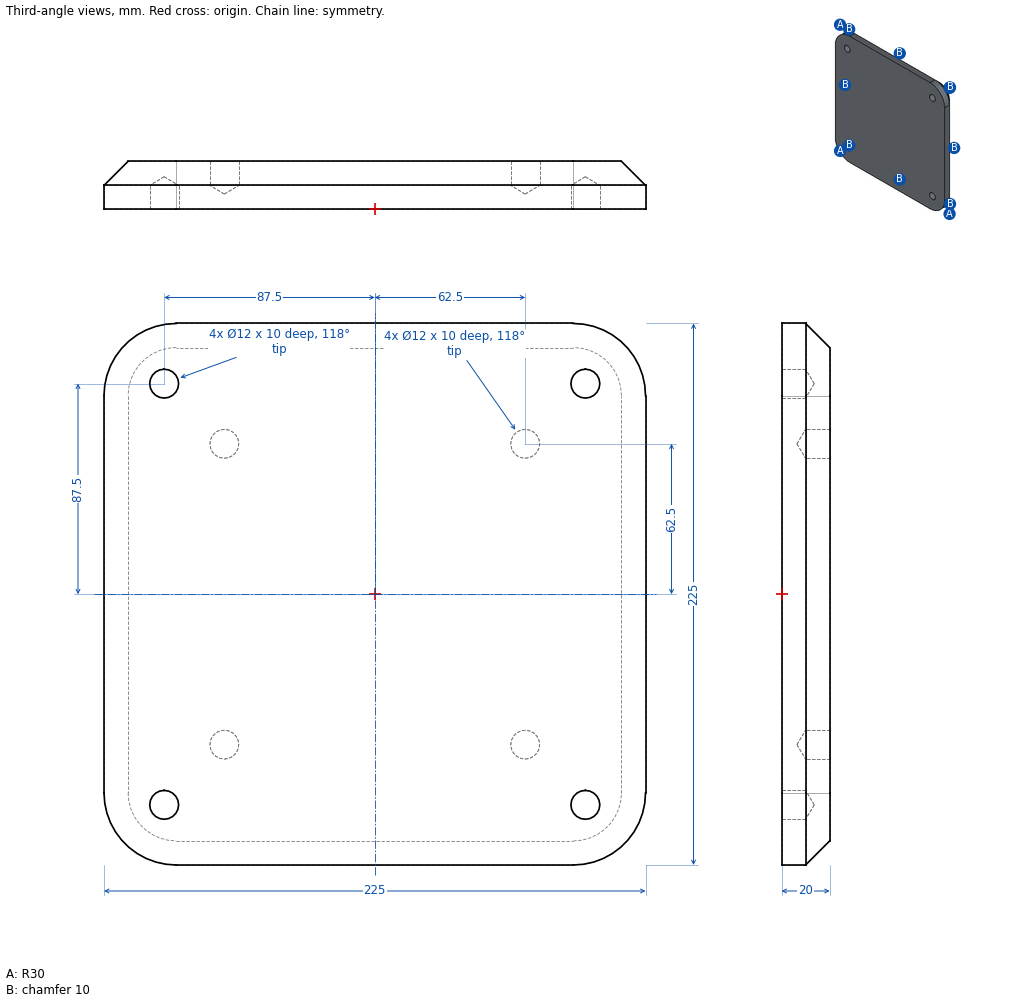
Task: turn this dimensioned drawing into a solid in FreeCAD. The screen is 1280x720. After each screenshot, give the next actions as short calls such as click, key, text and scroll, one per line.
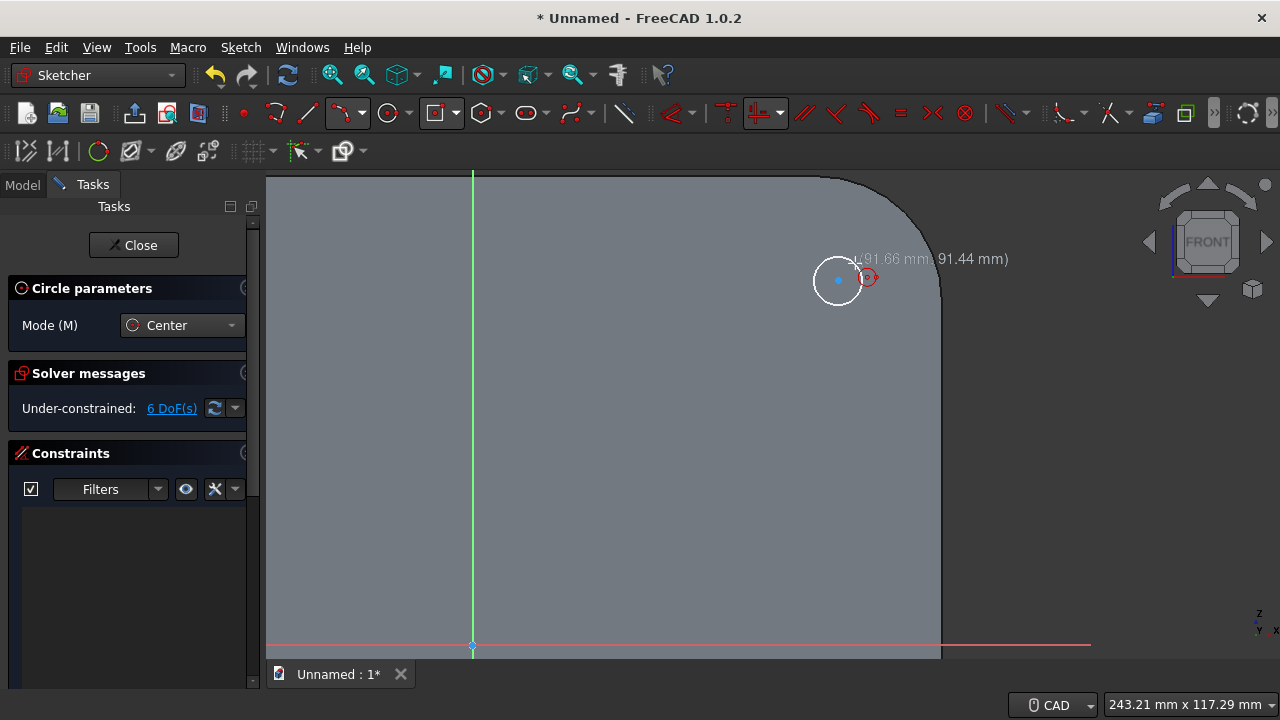
scroll(839, 280, down, 5)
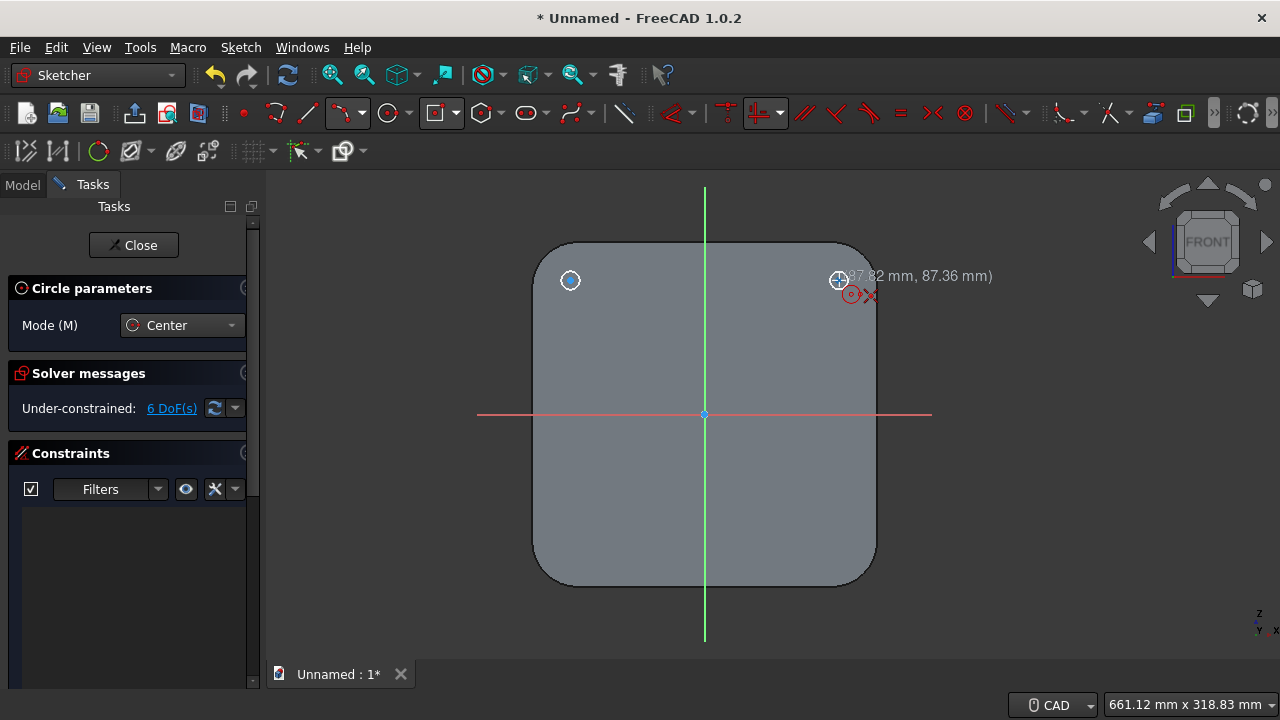
scroll(839, 549, up, 5)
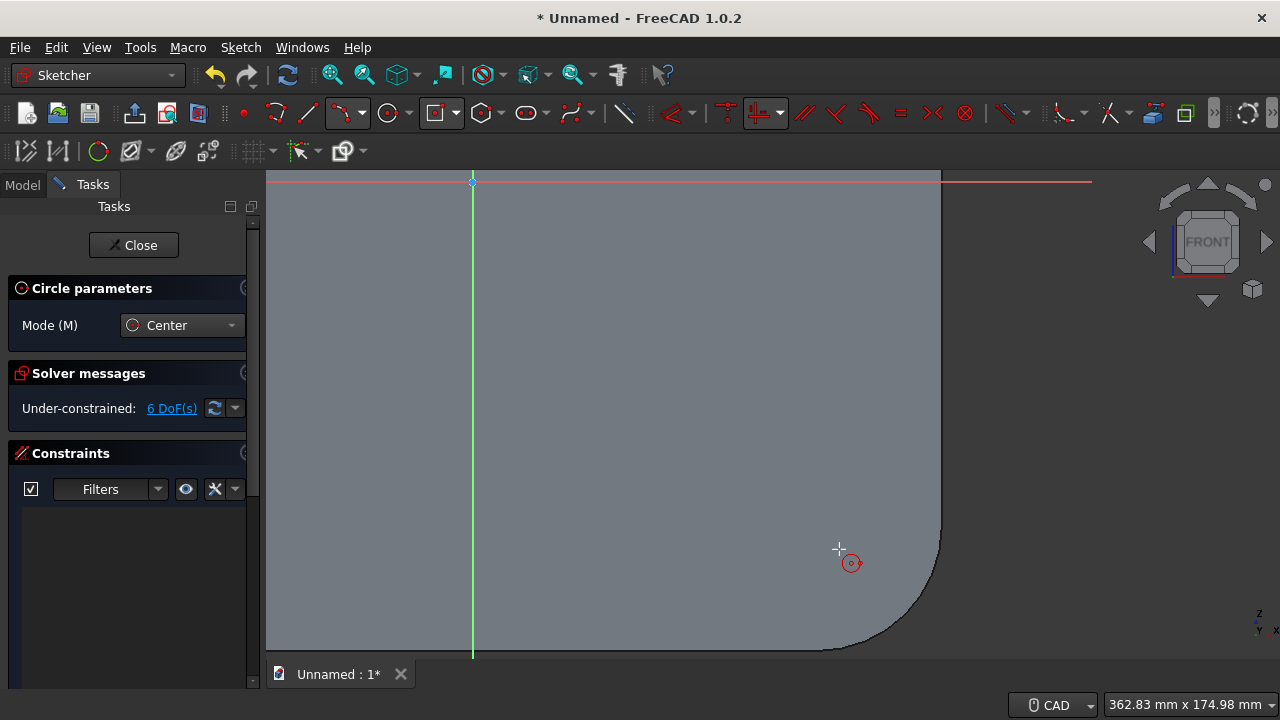
click(838, 547)
click(855, 529)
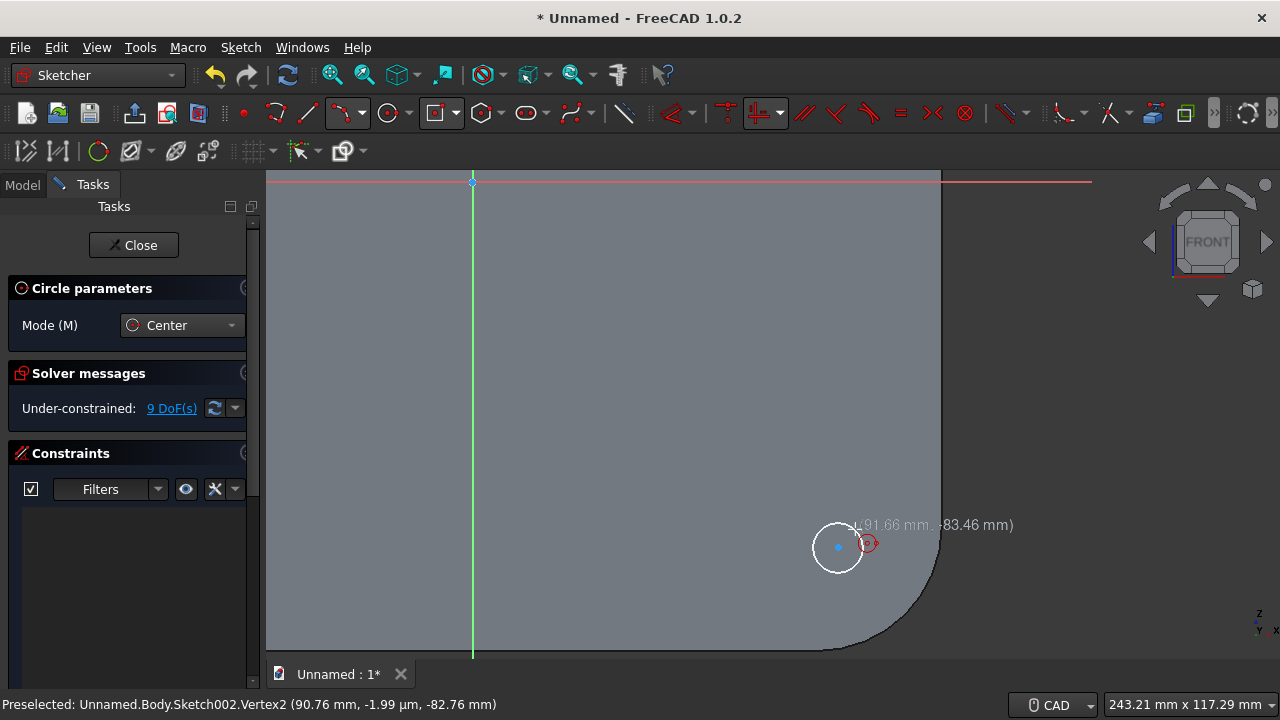
scroll(839, 550, down, 5)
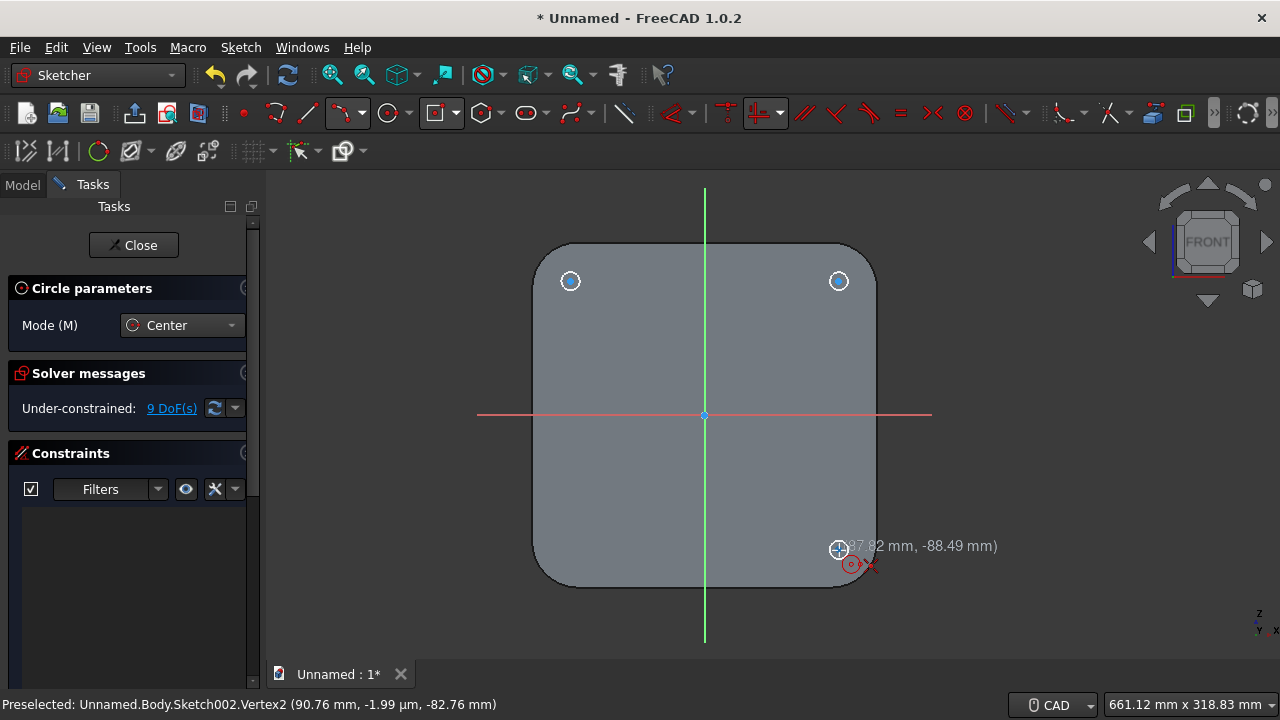
scroll(570, 549, up, 5)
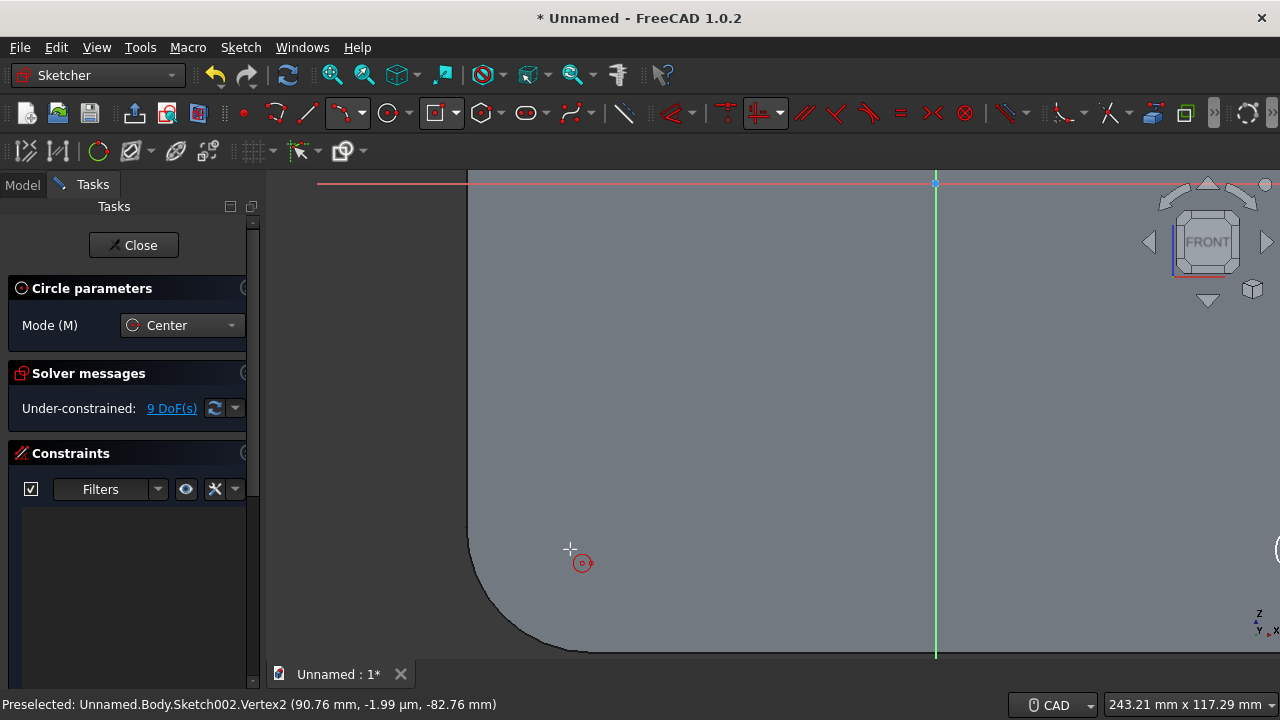
click(571, 549)
click(588, 531)
key(Escape)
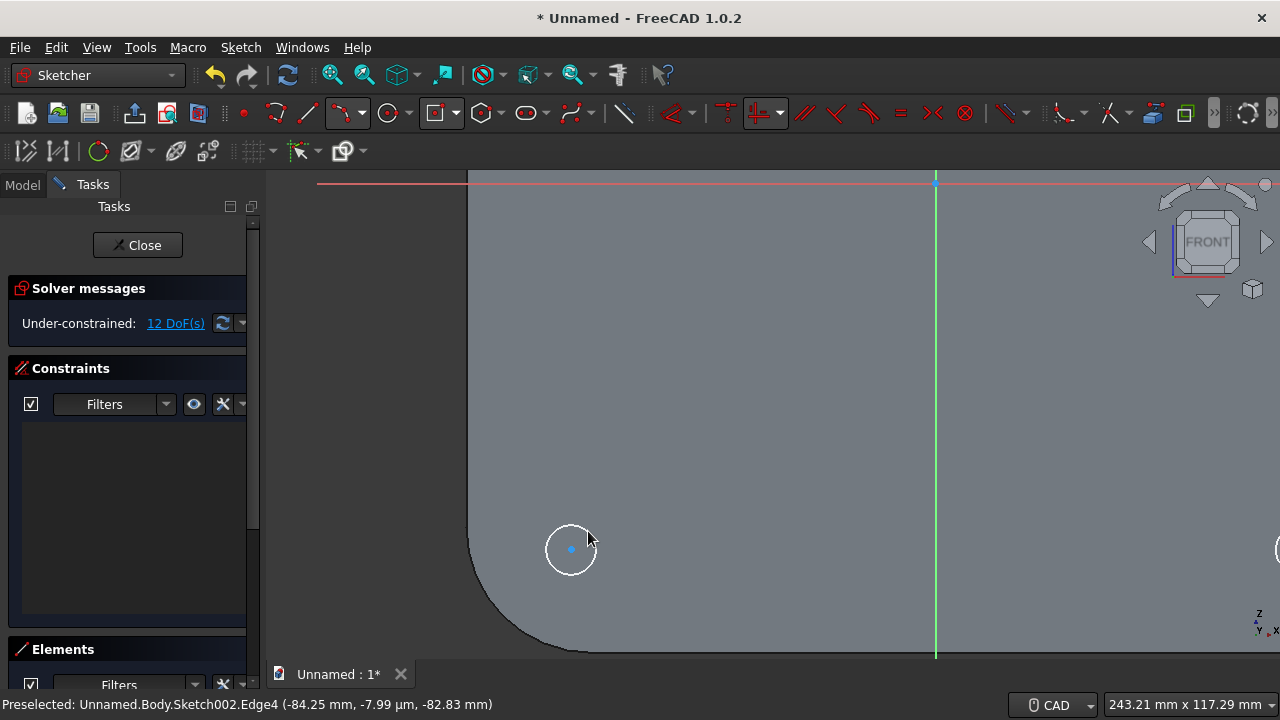
scroll(570, 549, down, 5)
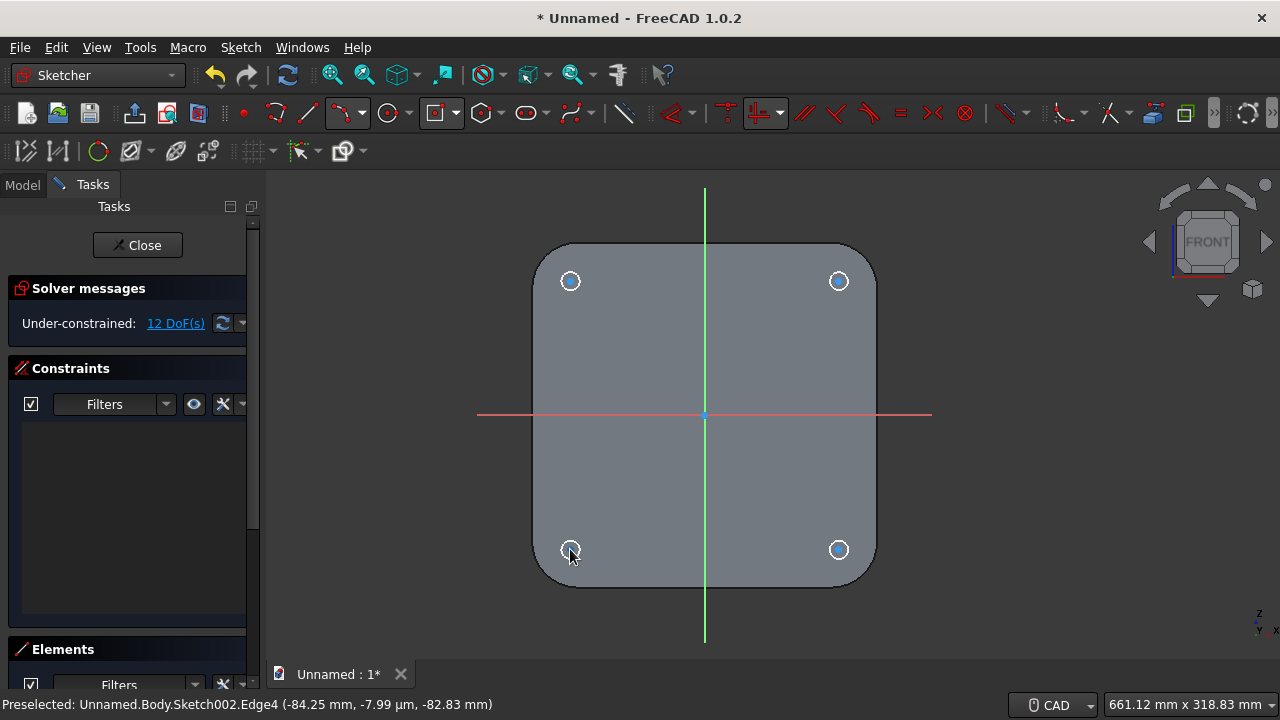
scroll(577, 275, up, 3)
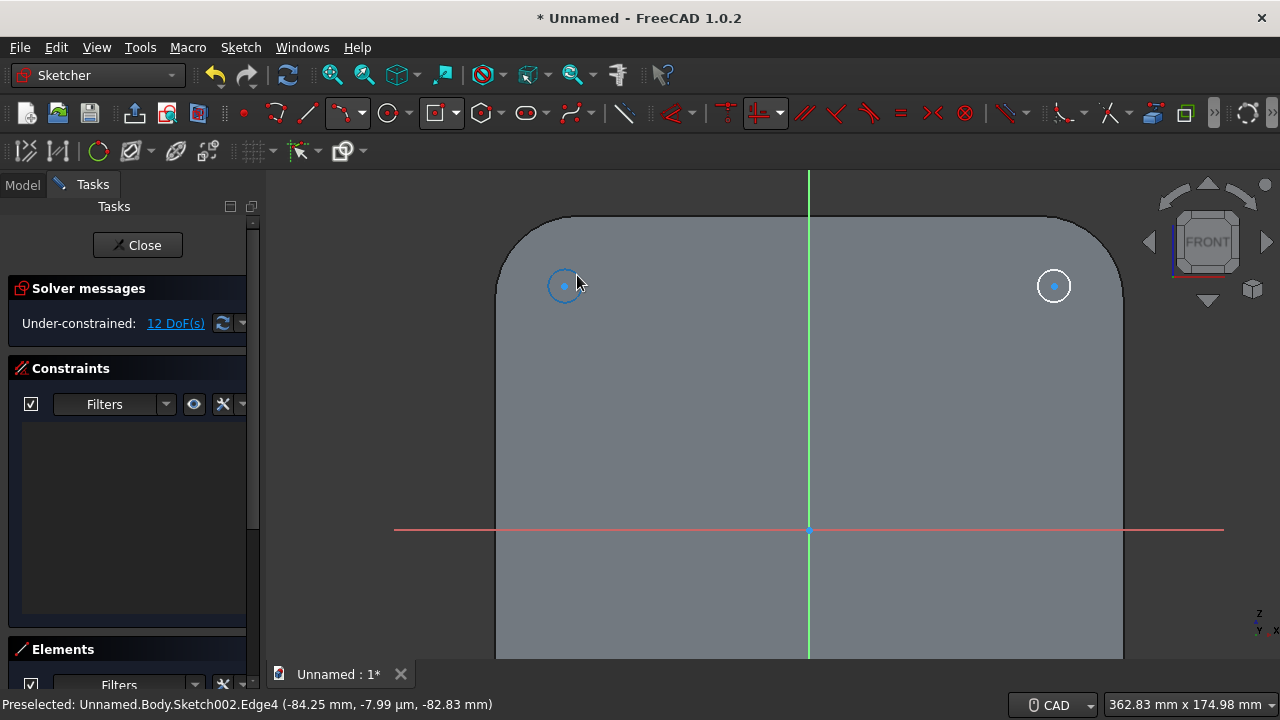
click(577, 274)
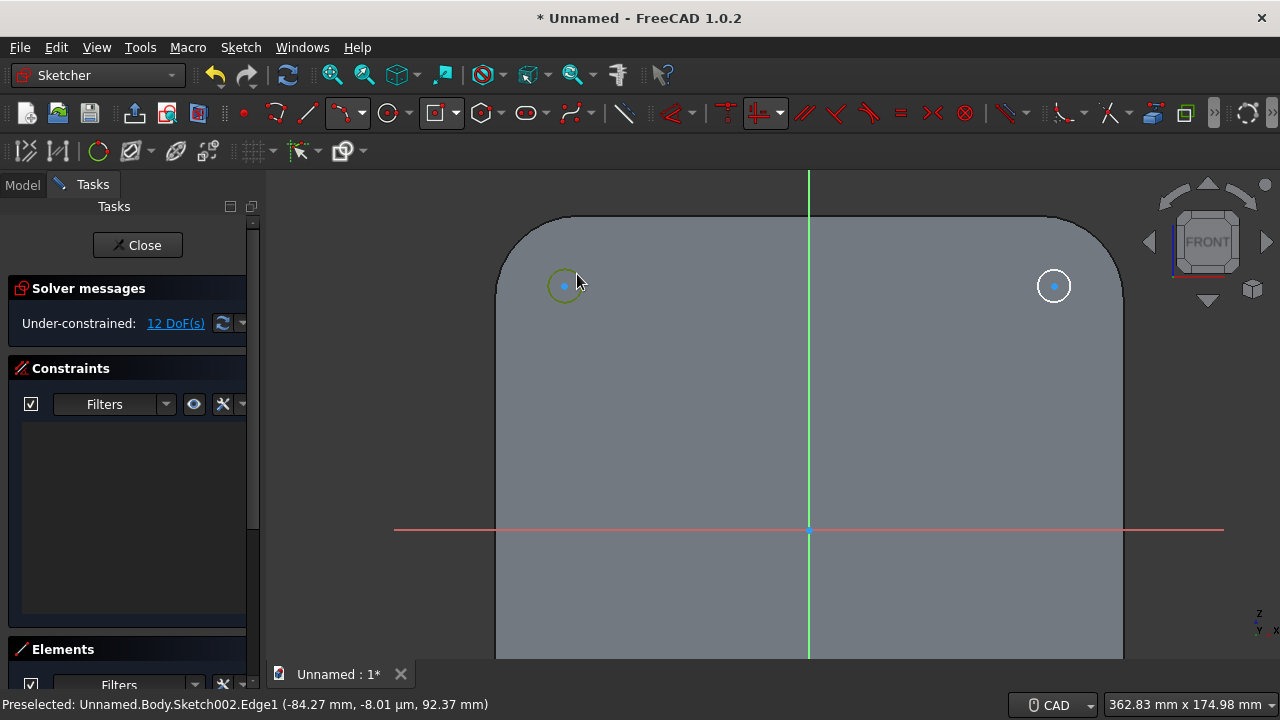
click(1065, 275)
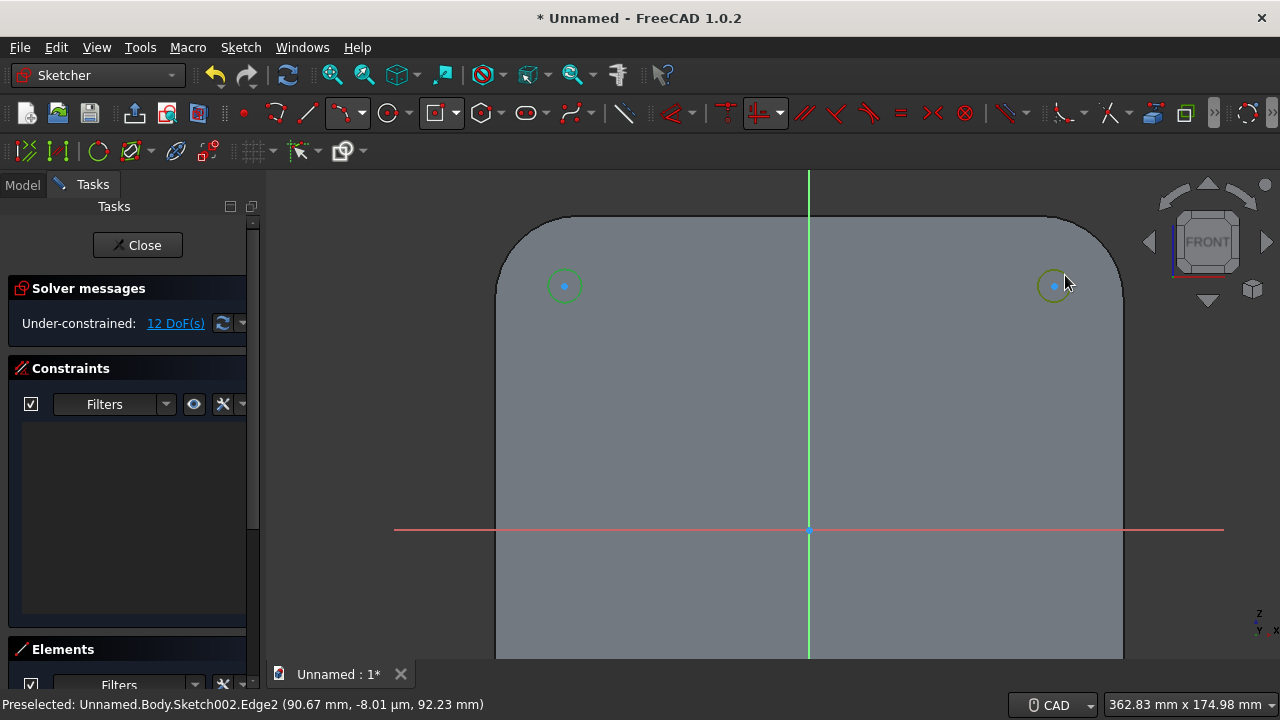
scroll(577, 274, down, 3)